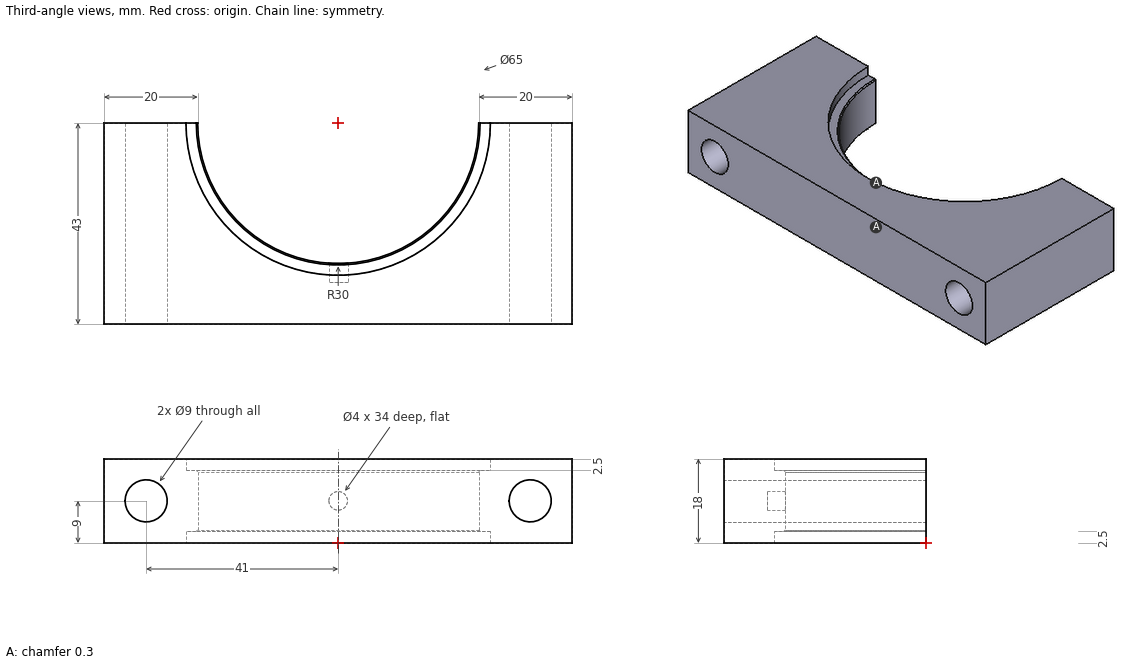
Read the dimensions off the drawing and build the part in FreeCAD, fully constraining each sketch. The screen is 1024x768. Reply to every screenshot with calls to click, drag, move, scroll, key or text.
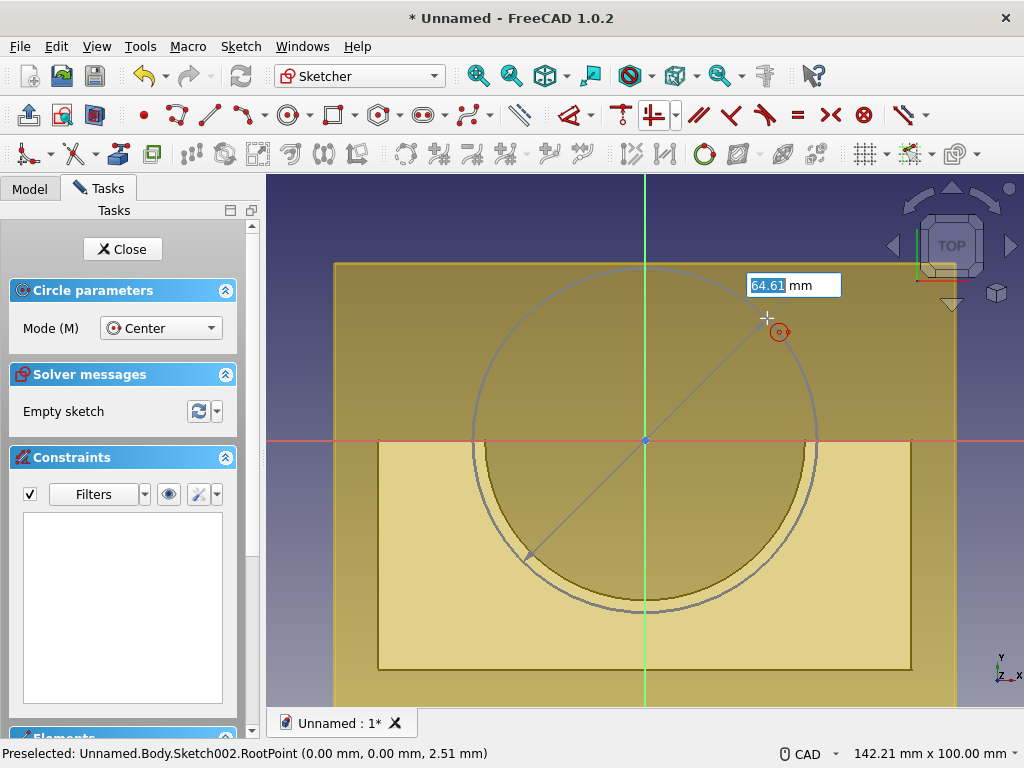
text(65)
key(Return)
key(Escape)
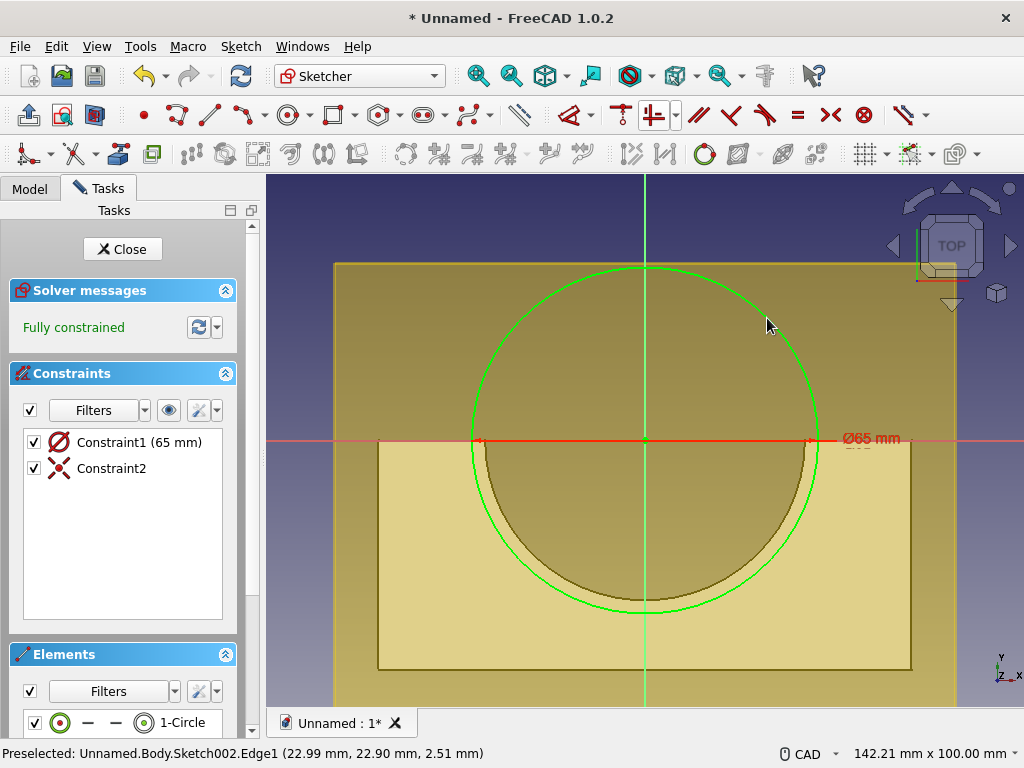
click(123, 249)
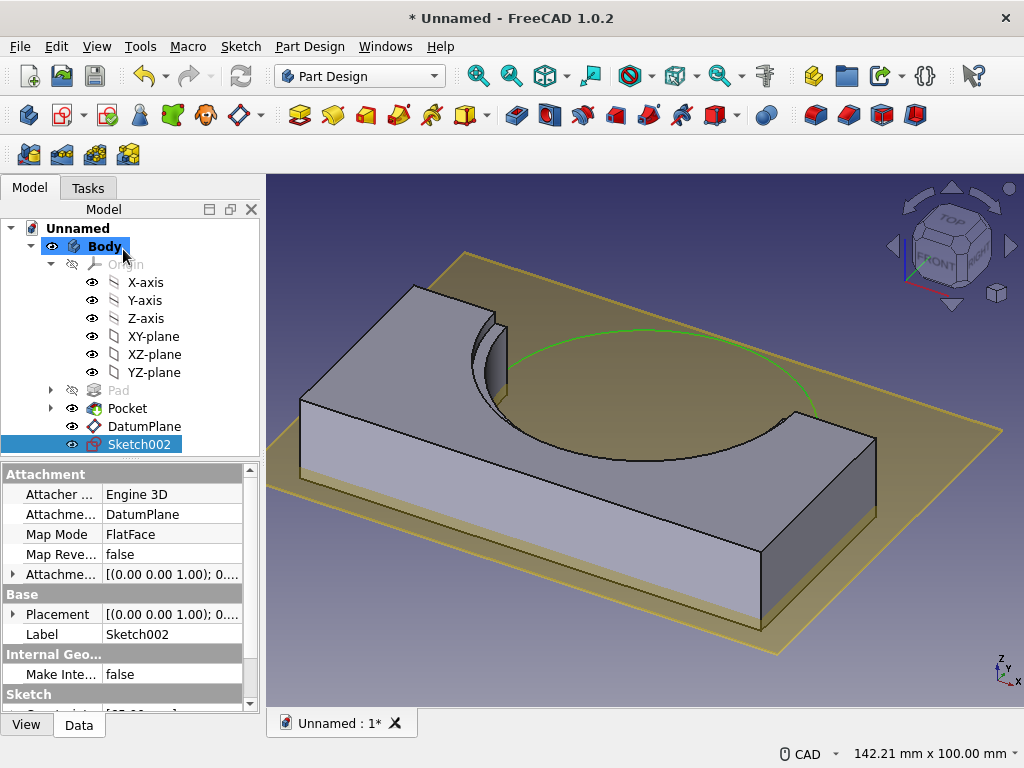
click(517, 116)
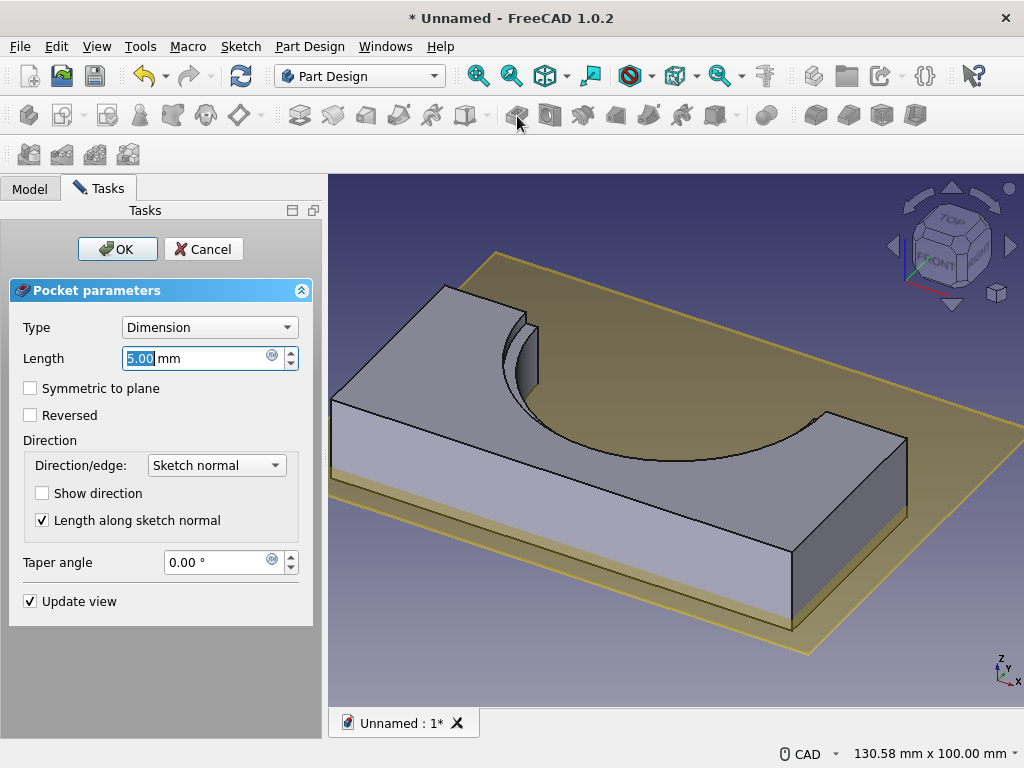
text(2.5)
key(Tab)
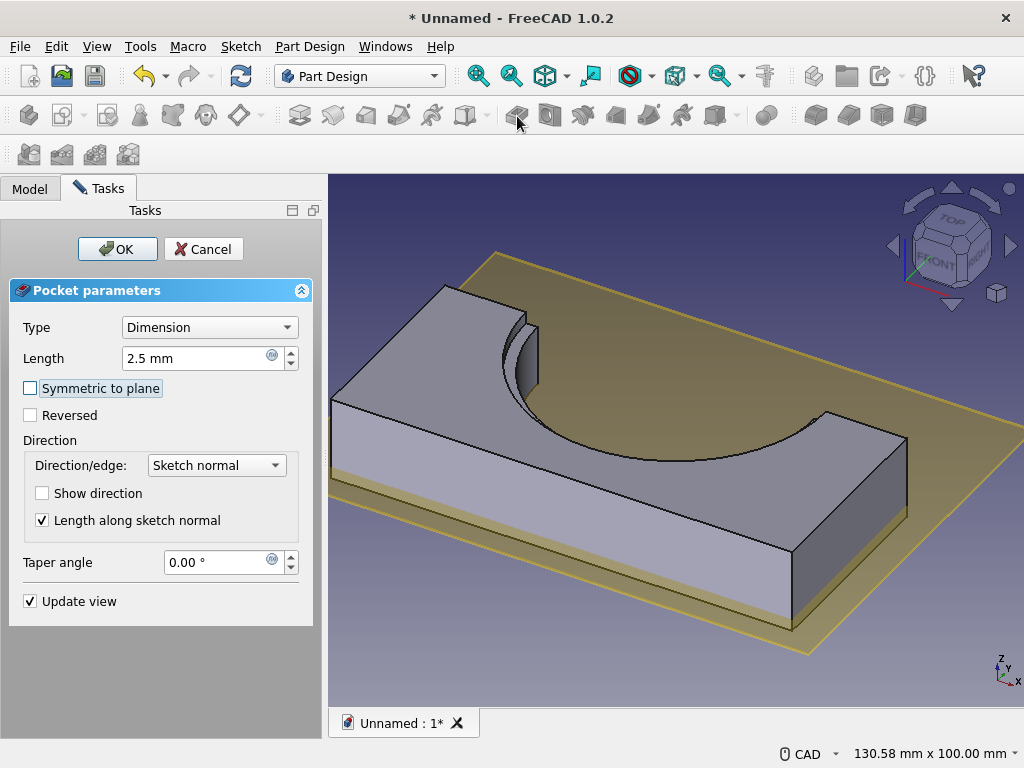
click(118, 249)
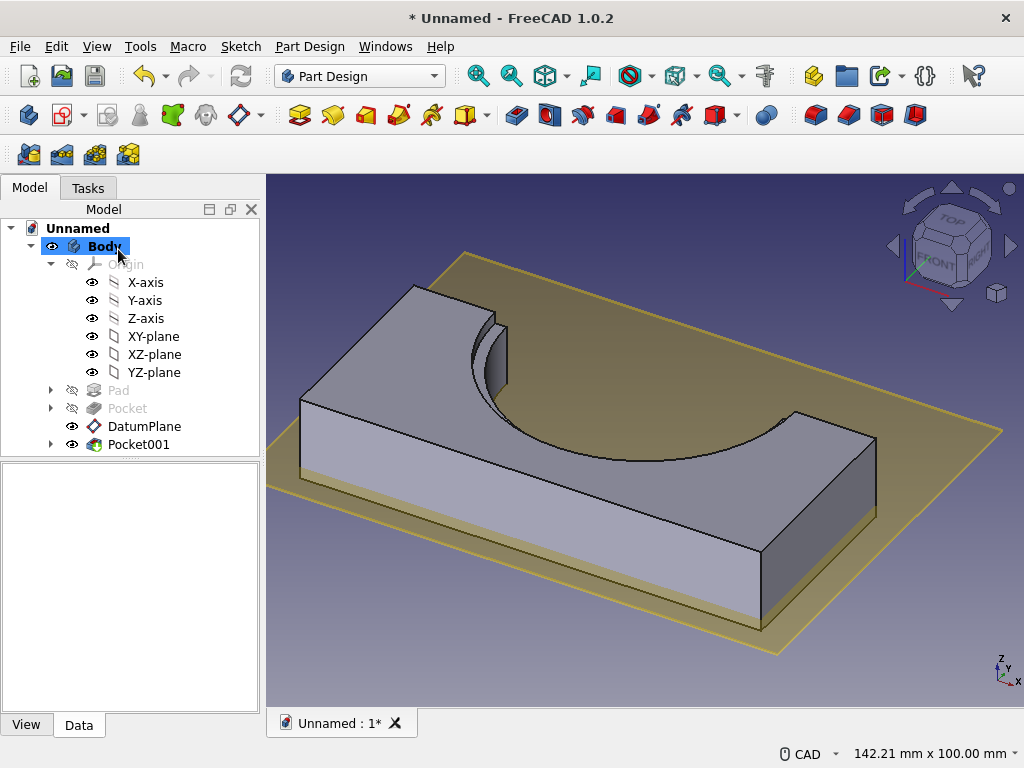
click(117, 426)
key(space)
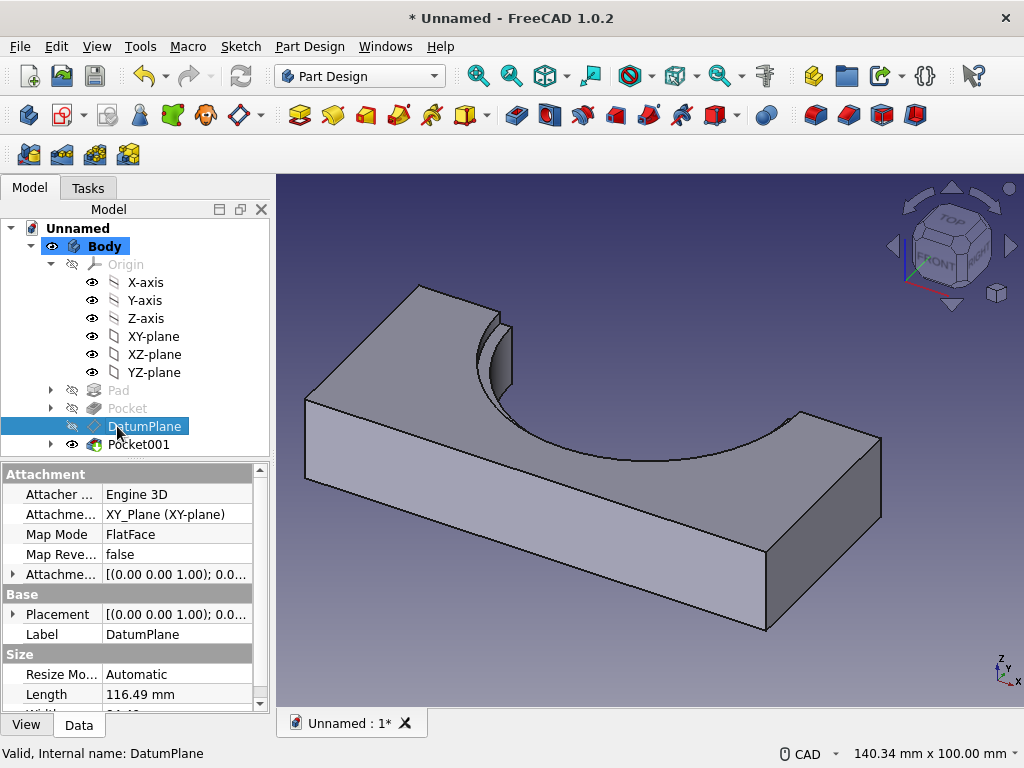
click(492, 358)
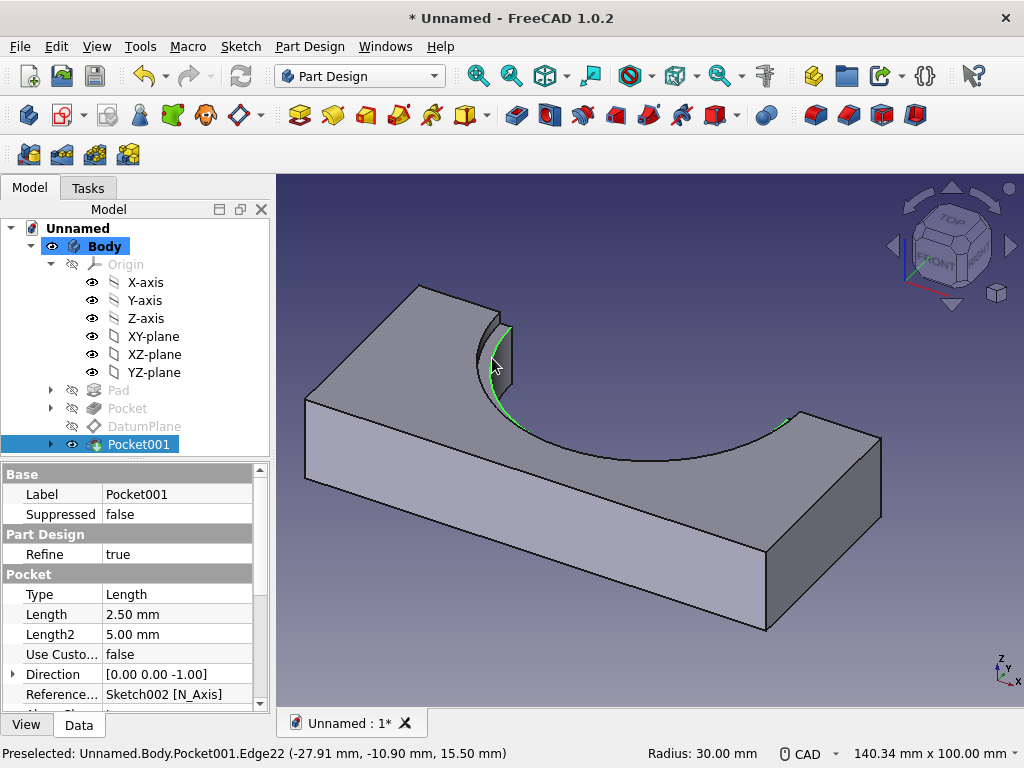
key(0)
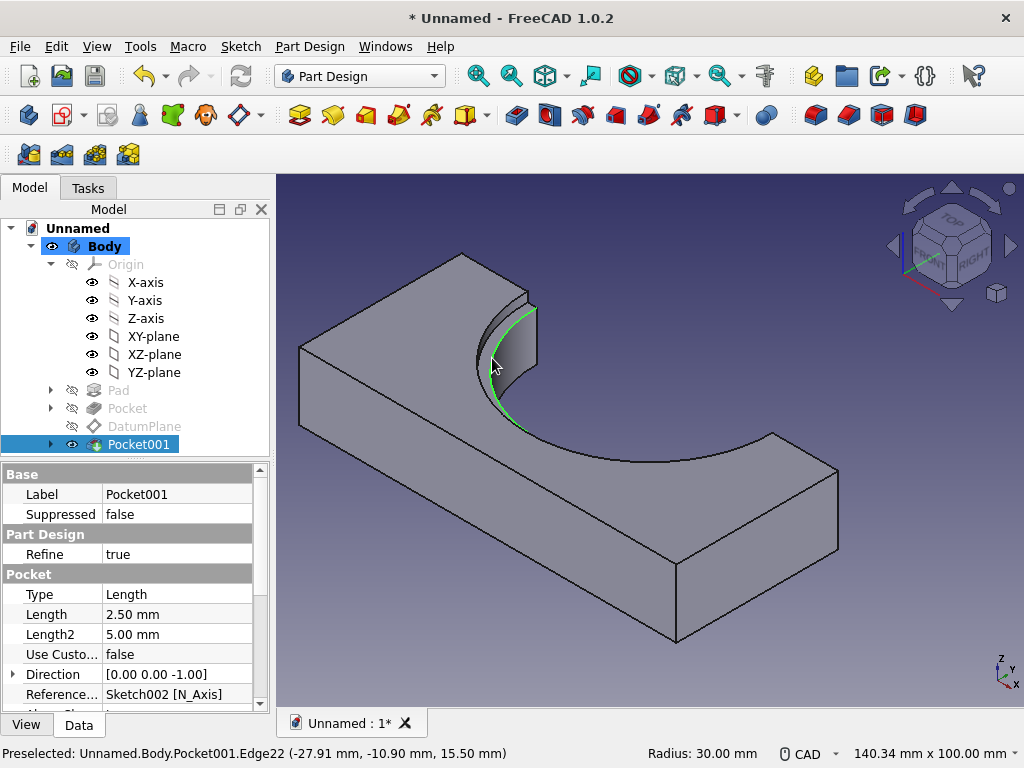
key(2)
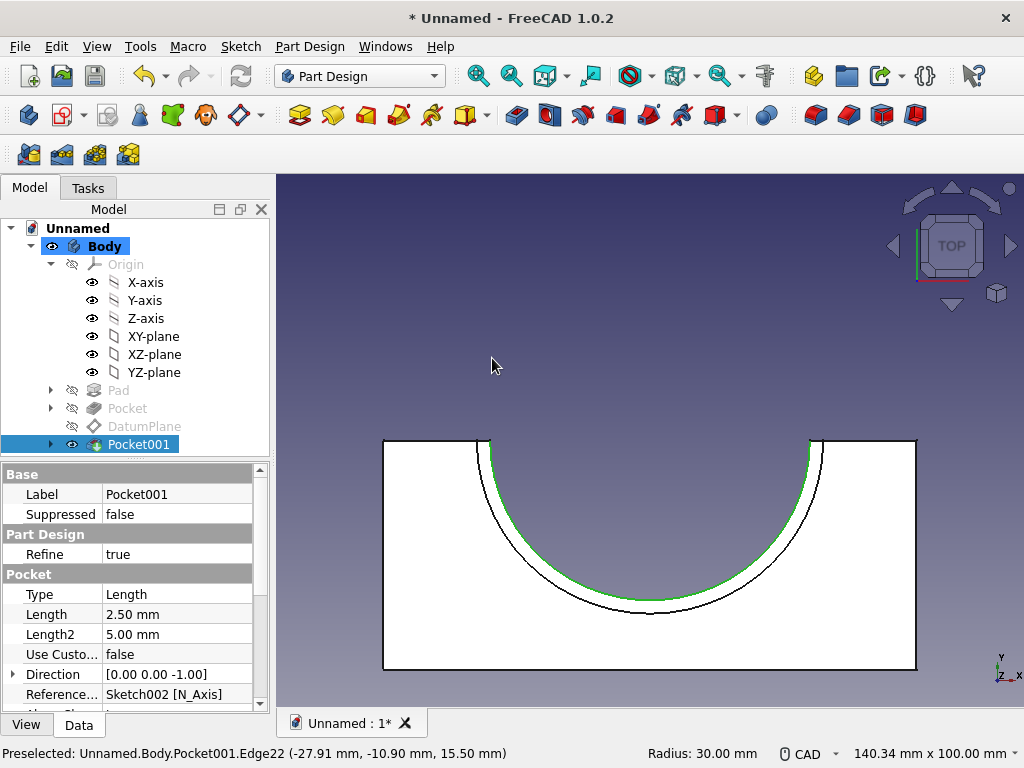
key(1)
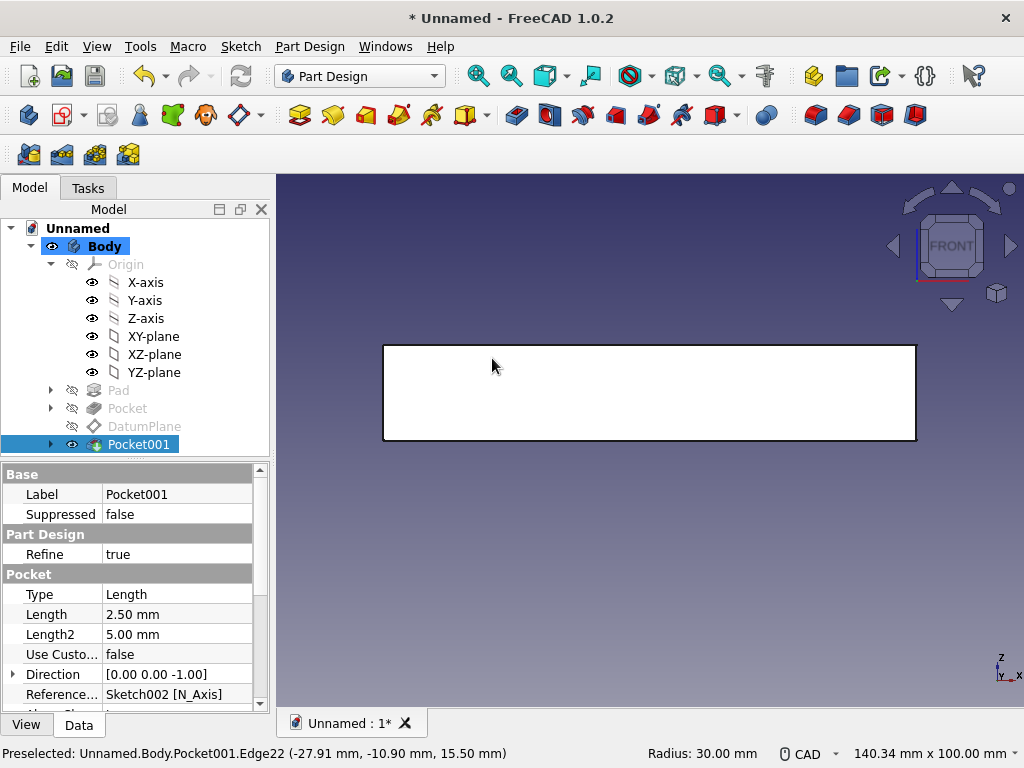
key(3)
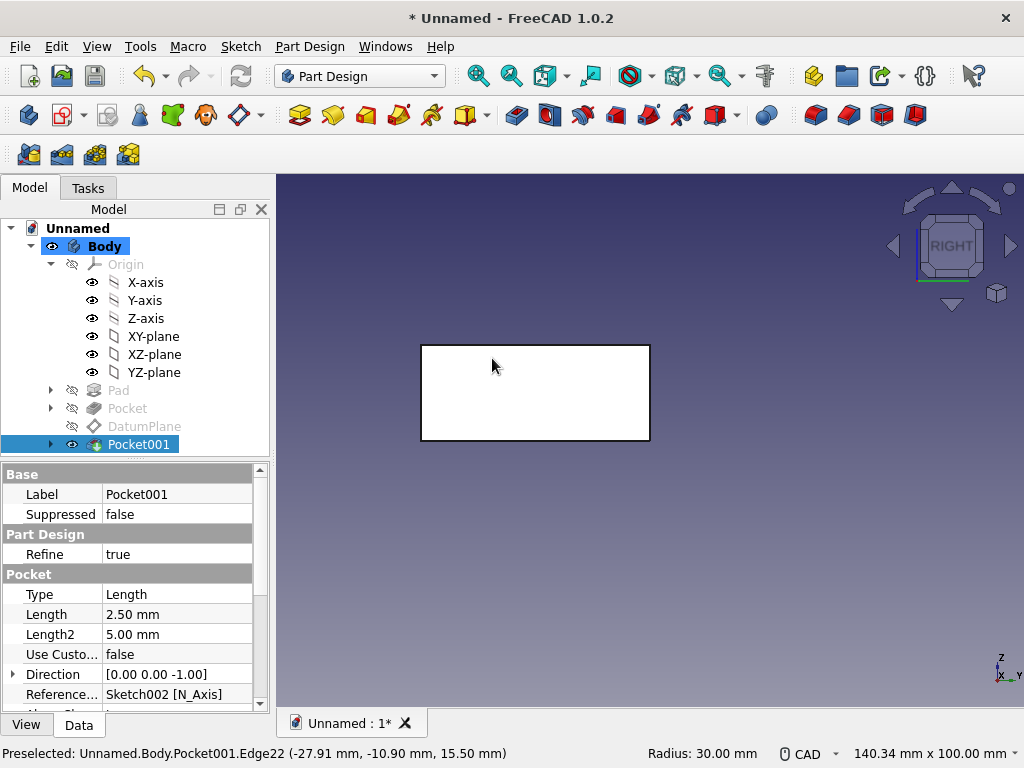
click(479, 76)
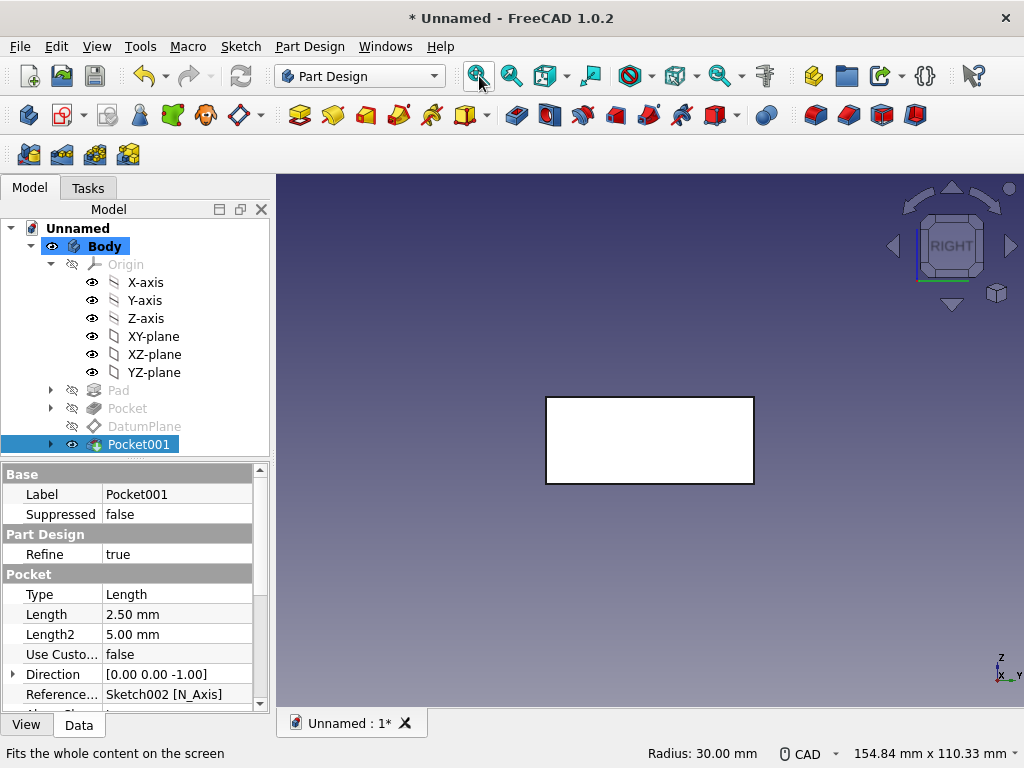
key(5)